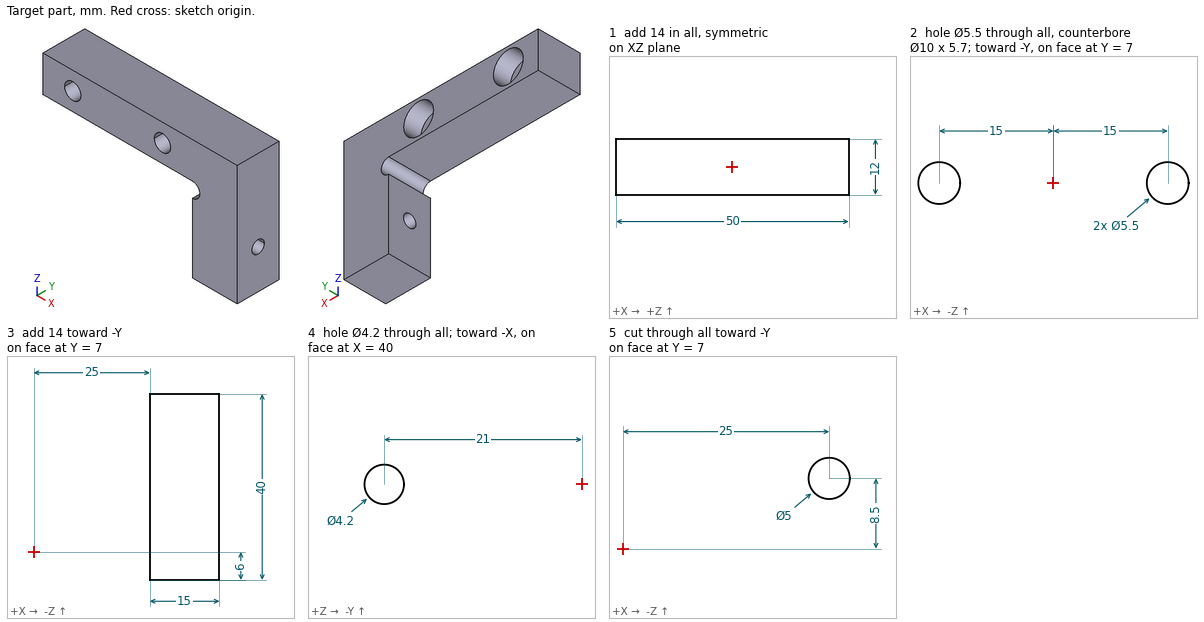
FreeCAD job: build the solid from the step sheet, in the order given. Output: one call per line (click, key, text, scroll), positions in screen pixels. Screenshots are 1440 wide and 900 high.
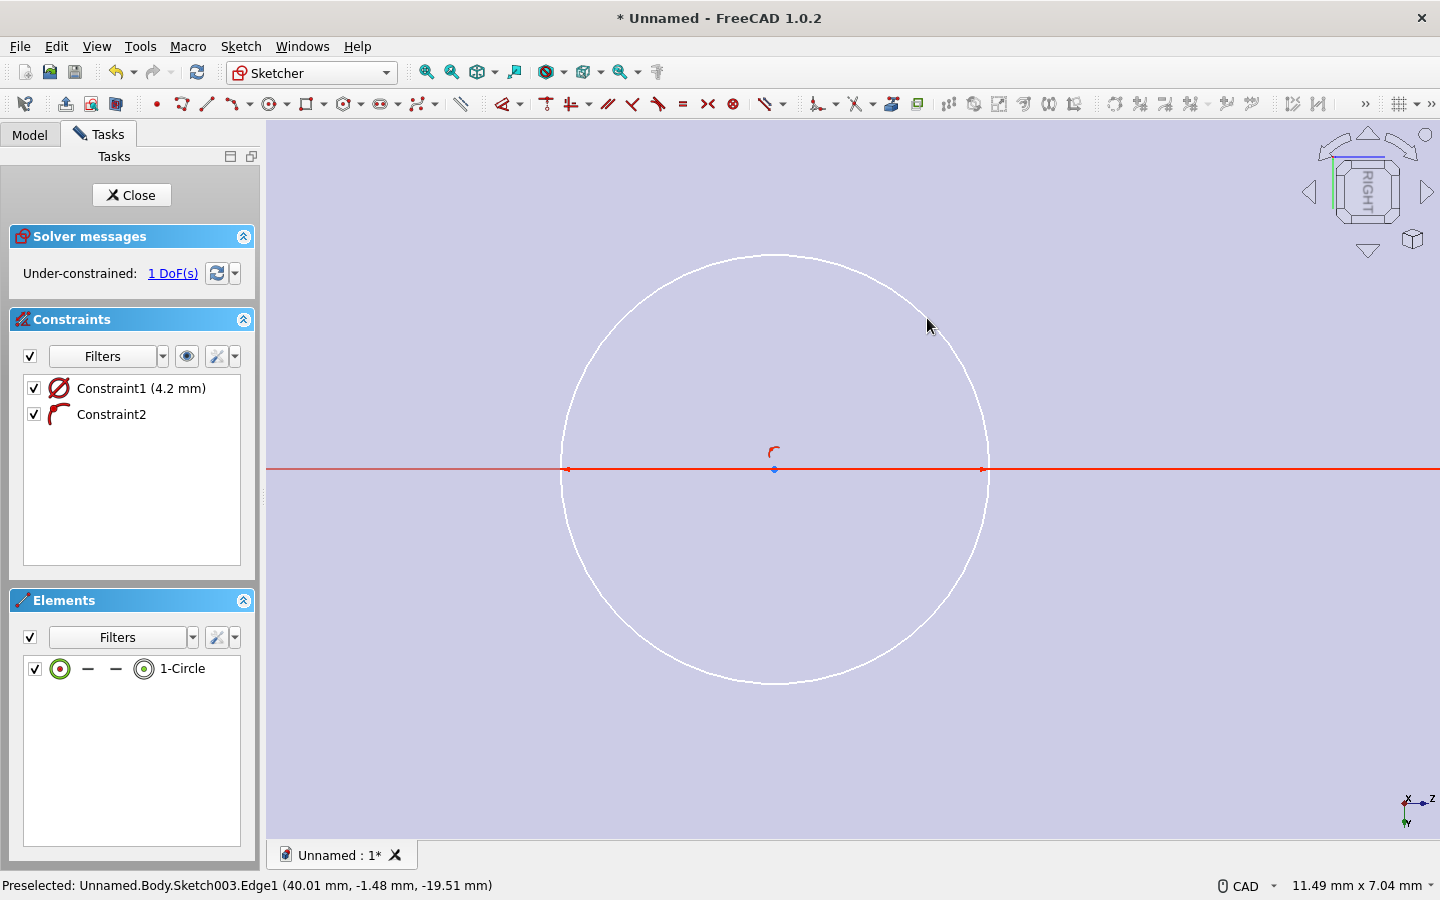
click(502, 104)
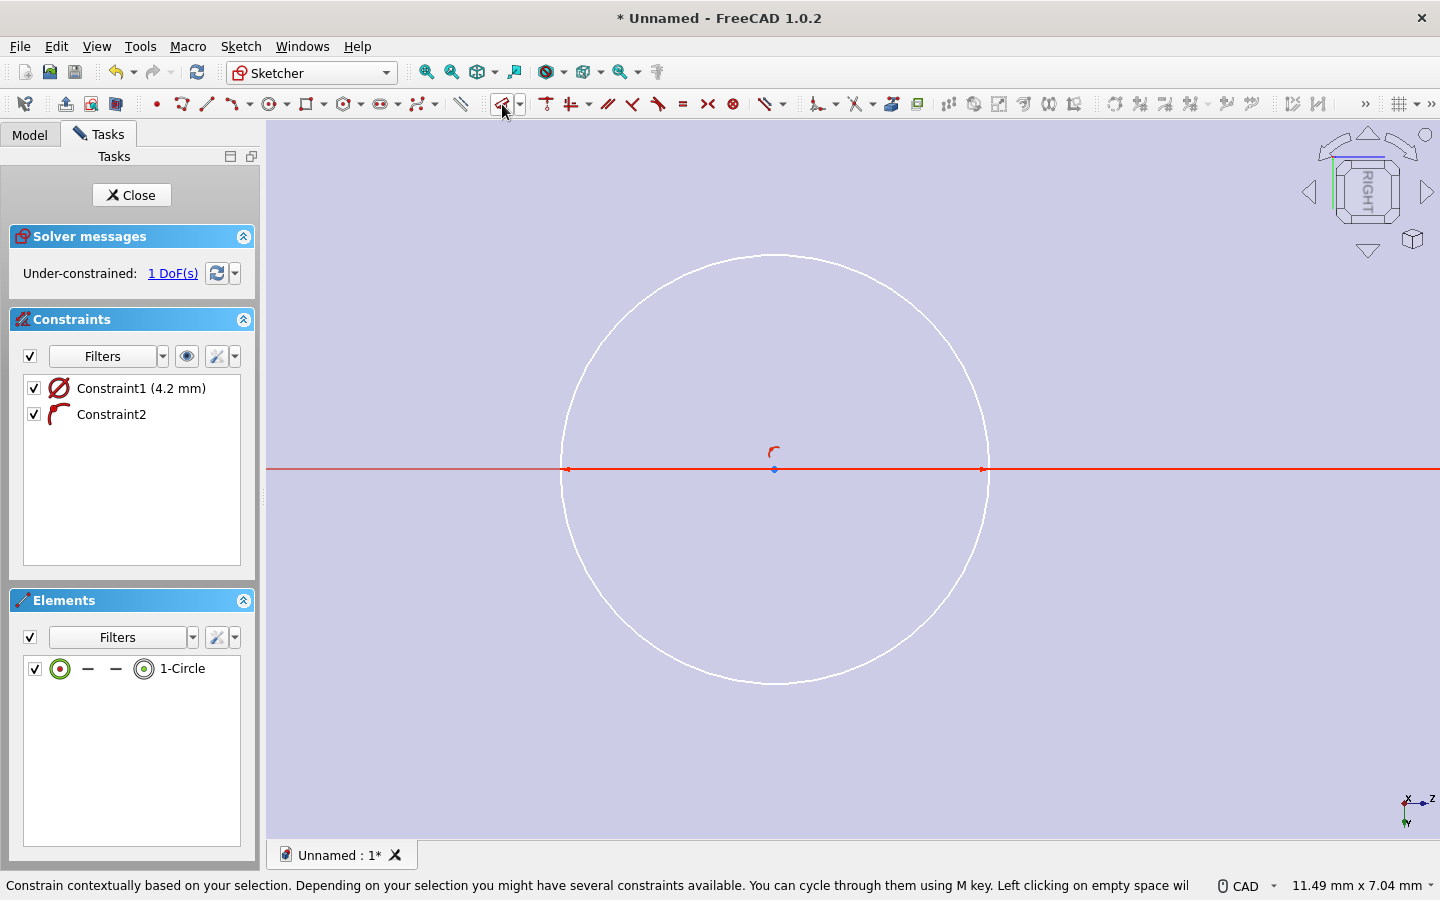
click(775, 469)
click(1025, 503)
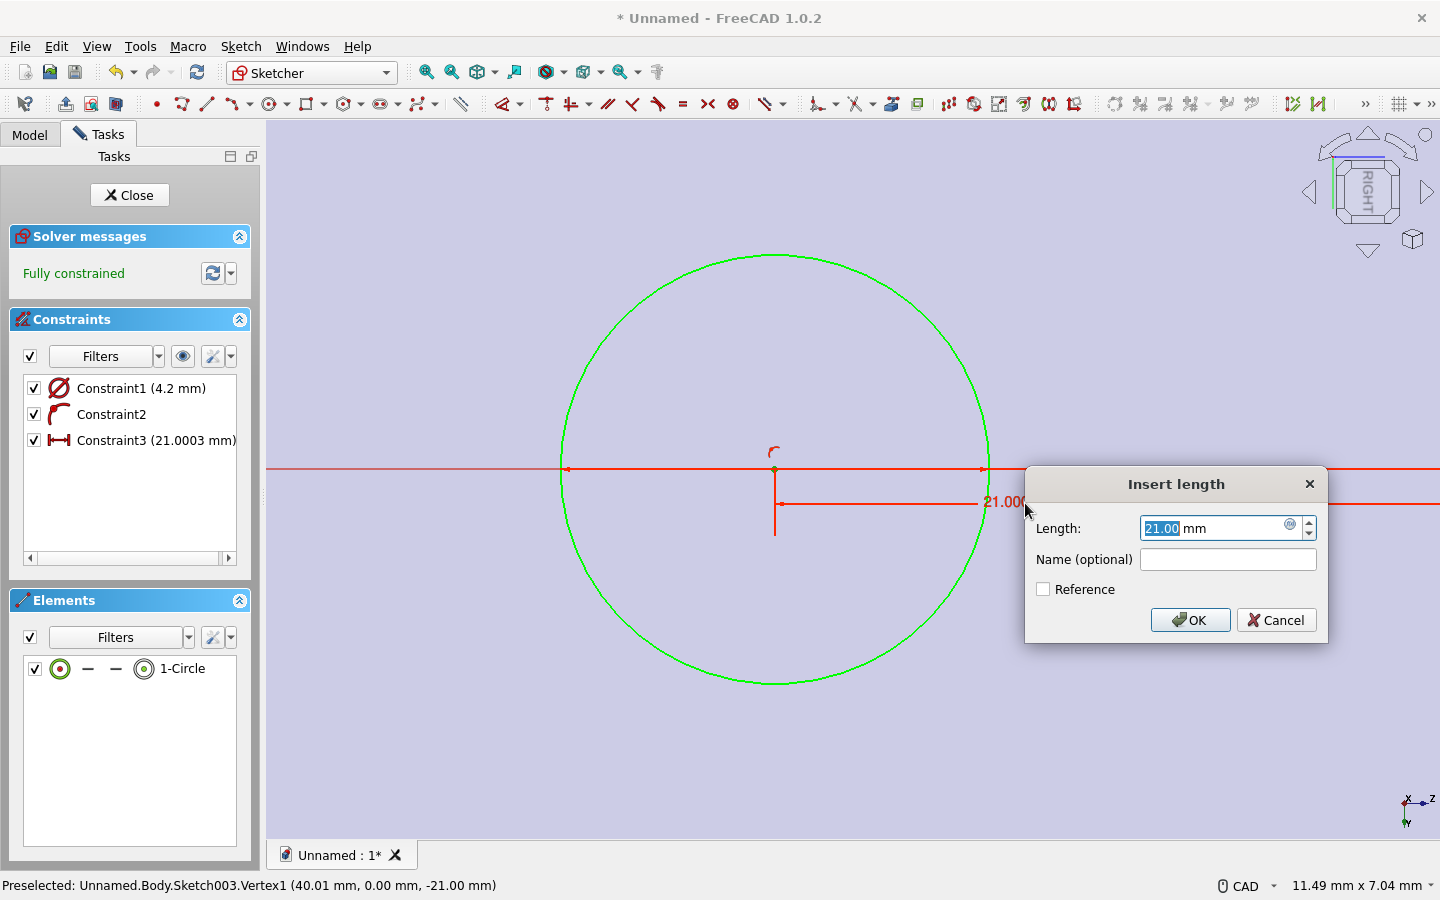
text(21)
key(Return)
key(Escape)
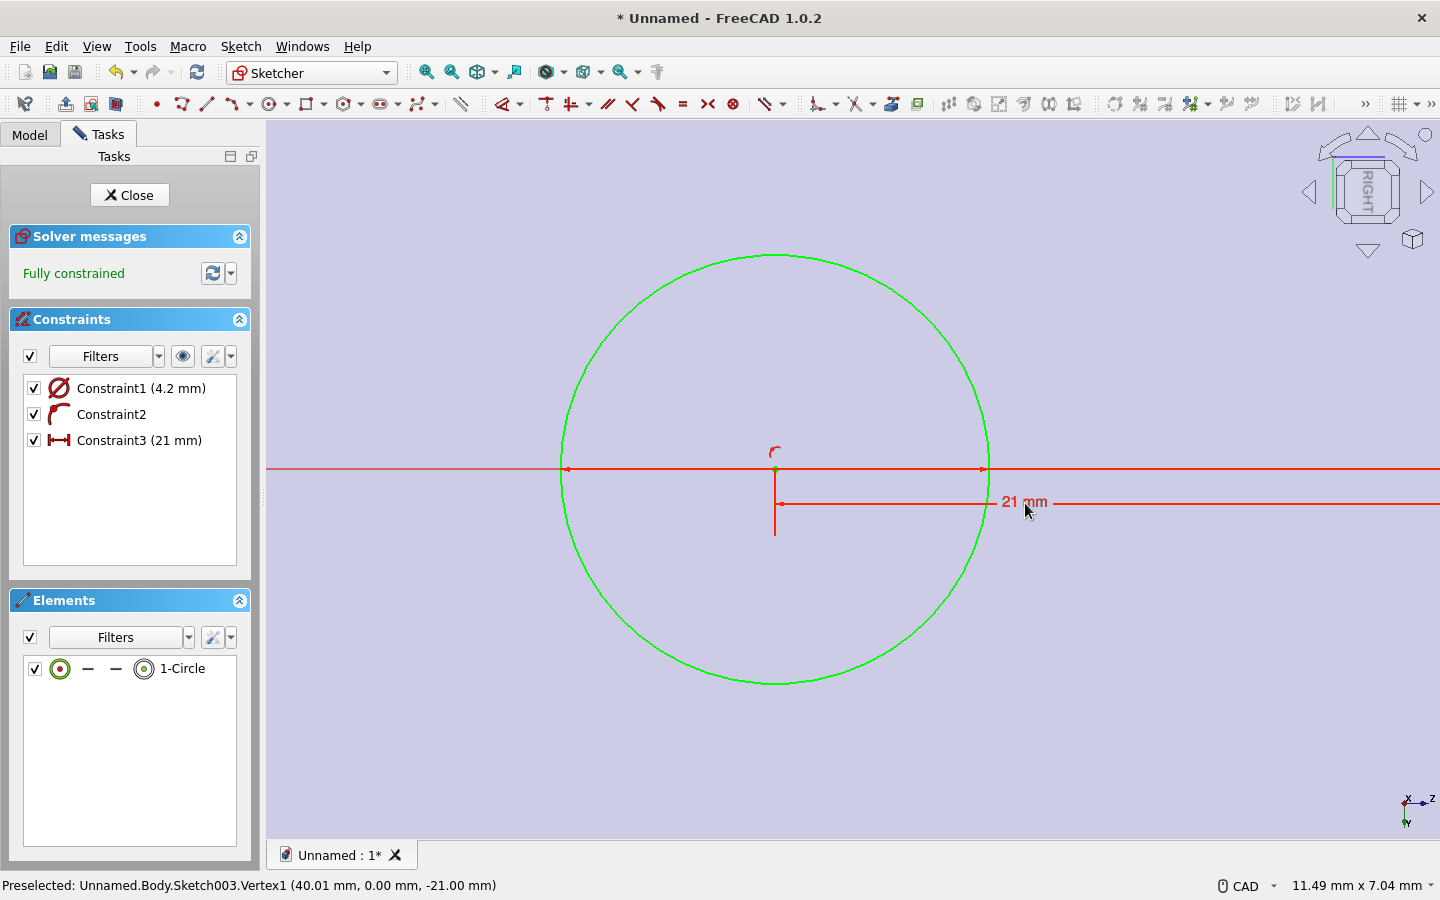
click(130, 195)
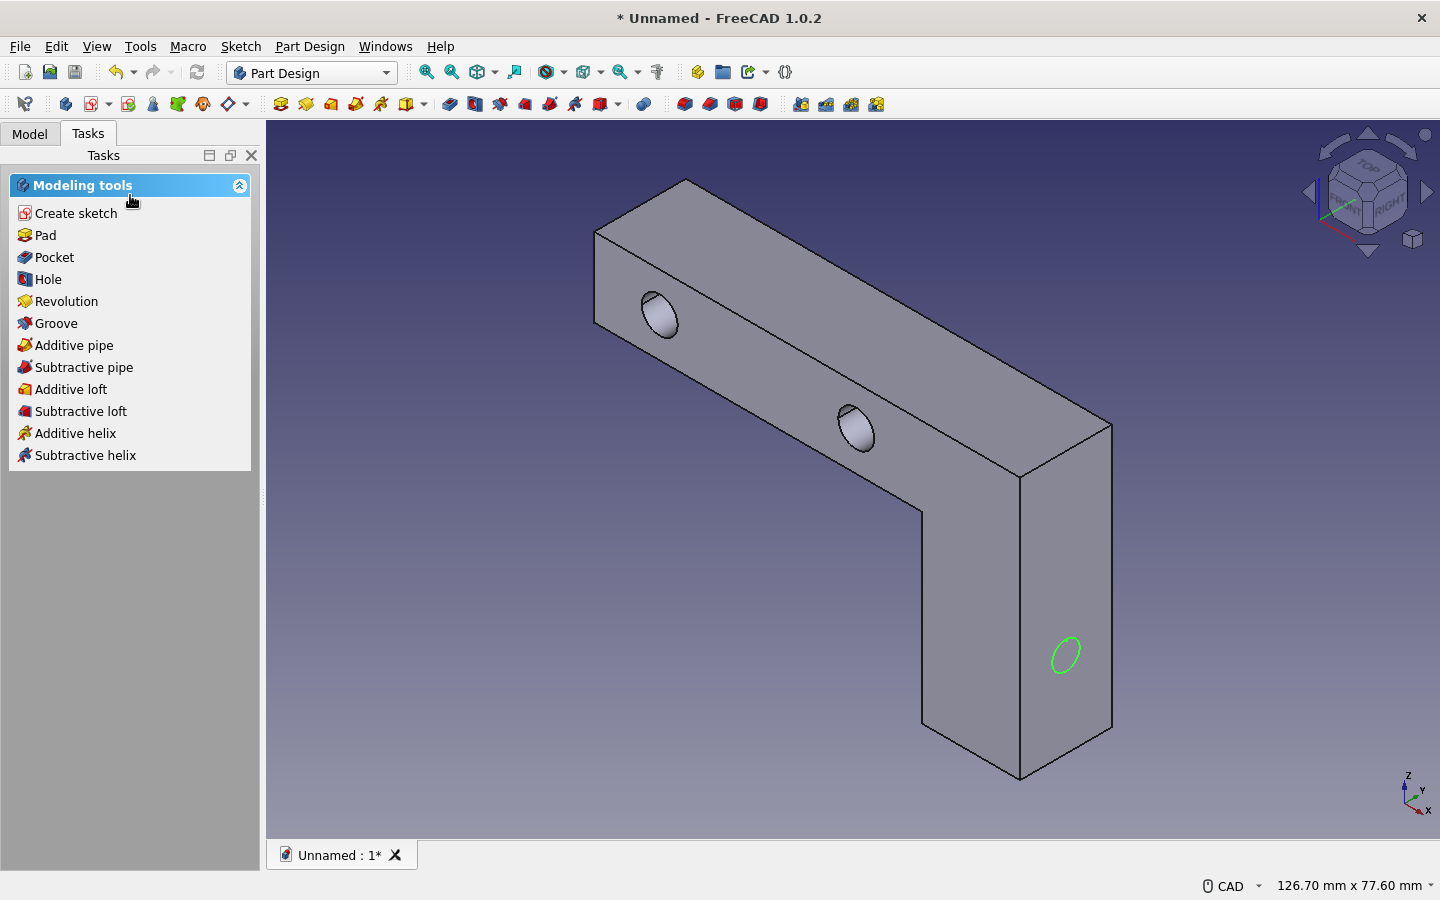
click(475, 104)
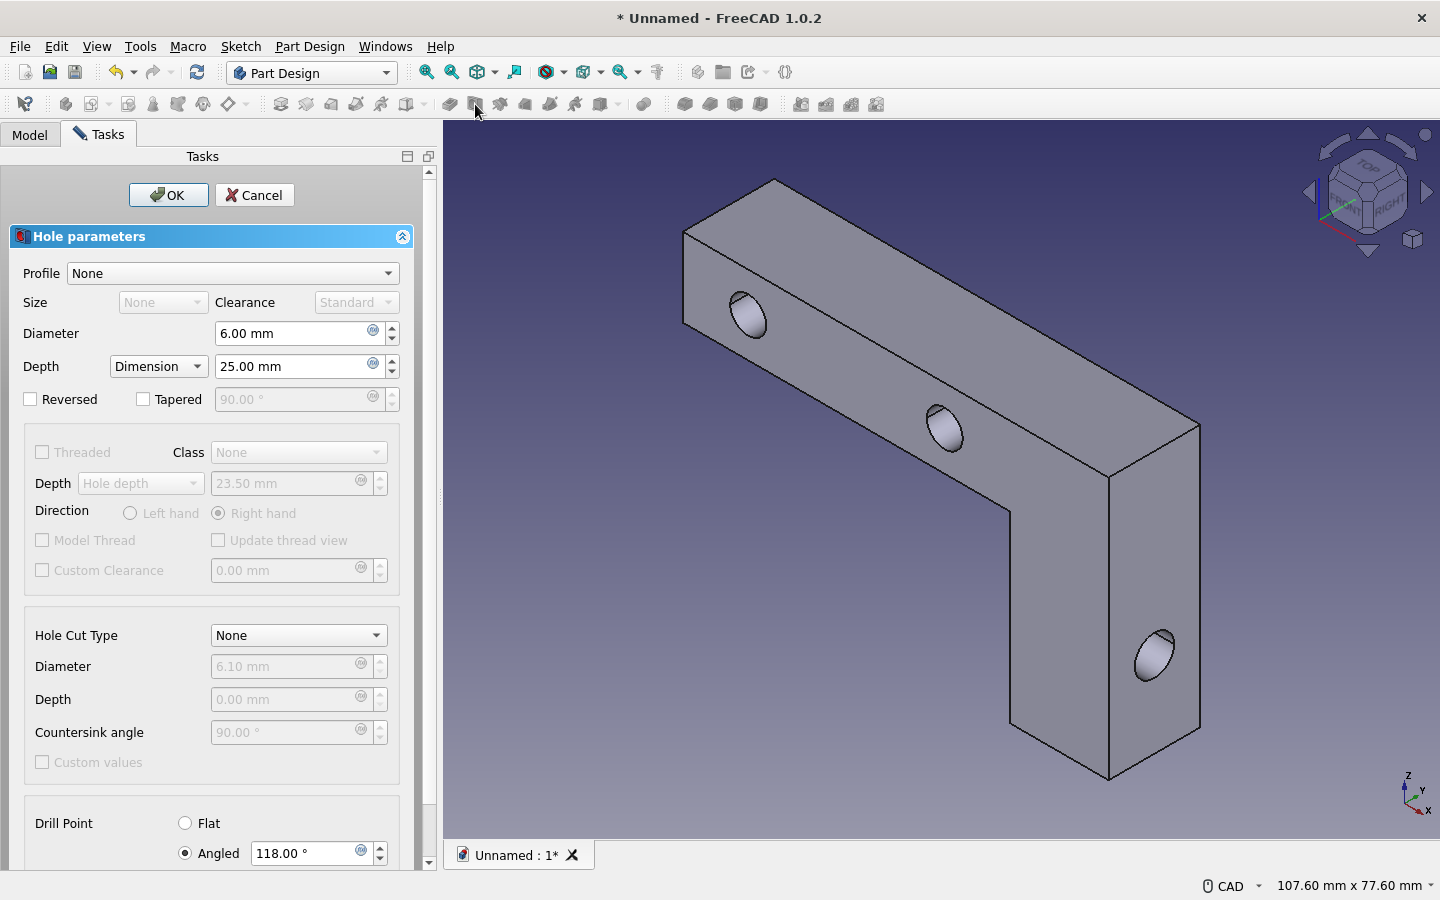
triple_click(300, 334)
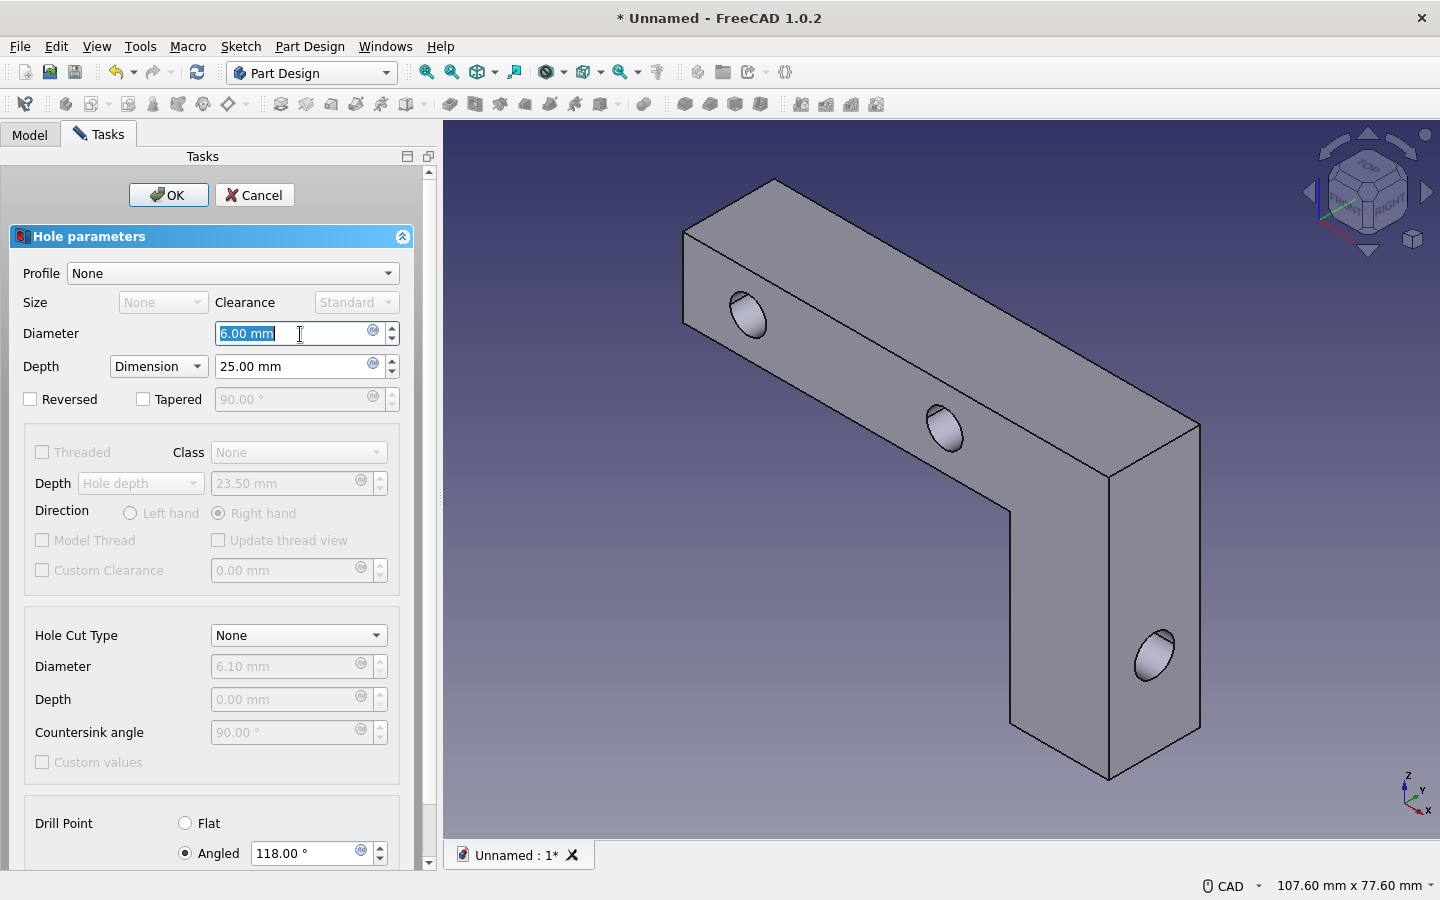
text(4.2)
key(Tab)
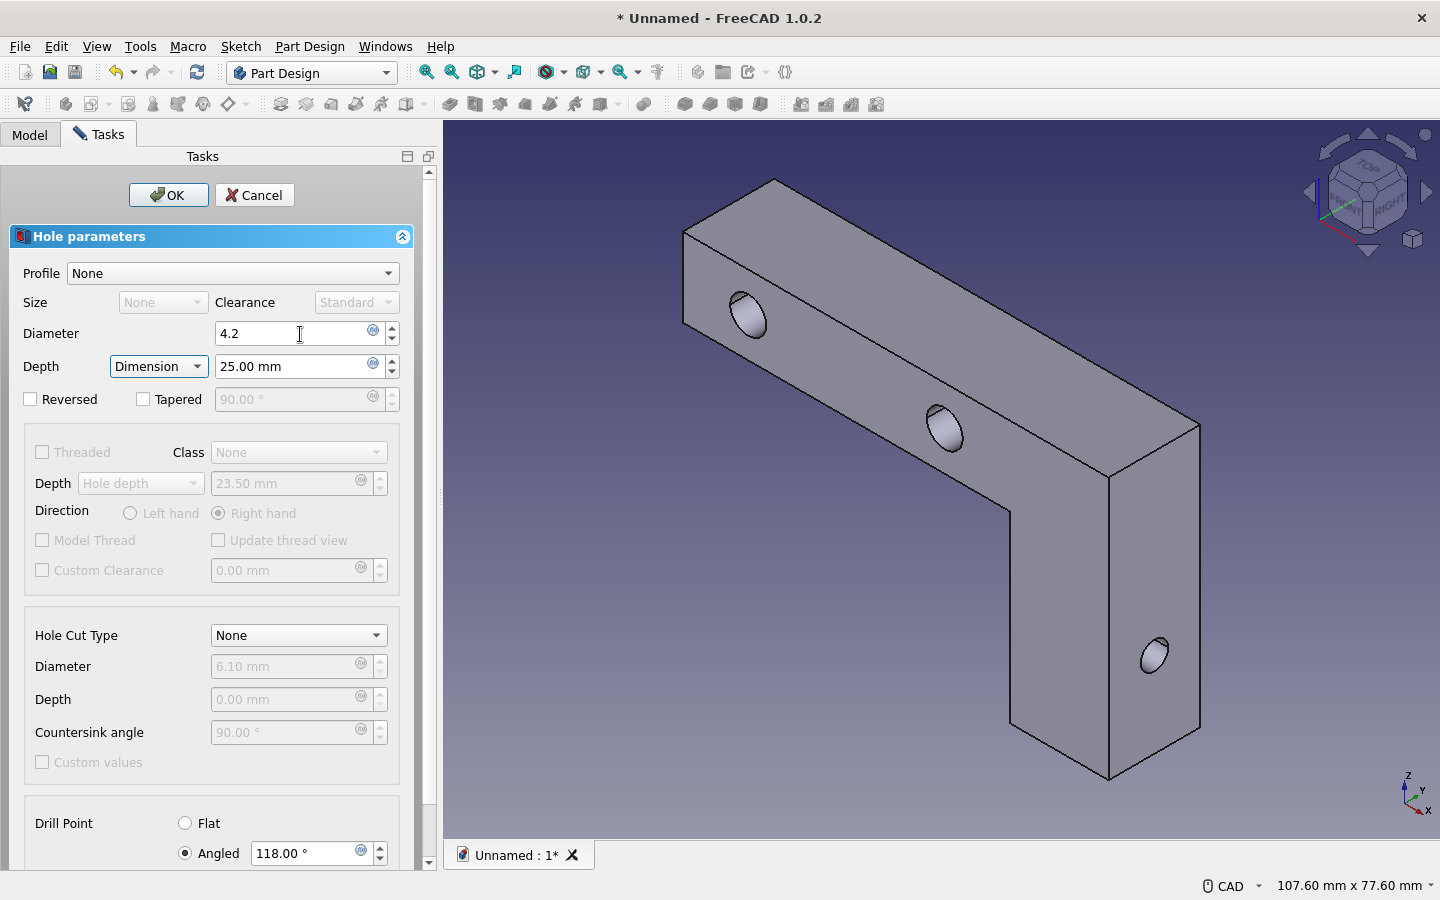
click(160, 366)